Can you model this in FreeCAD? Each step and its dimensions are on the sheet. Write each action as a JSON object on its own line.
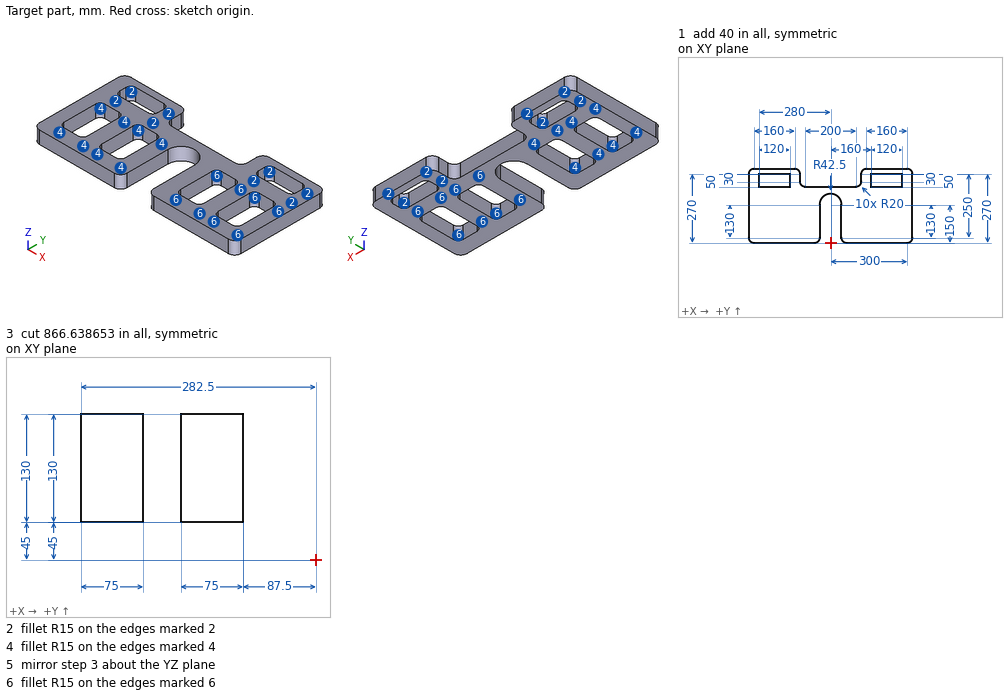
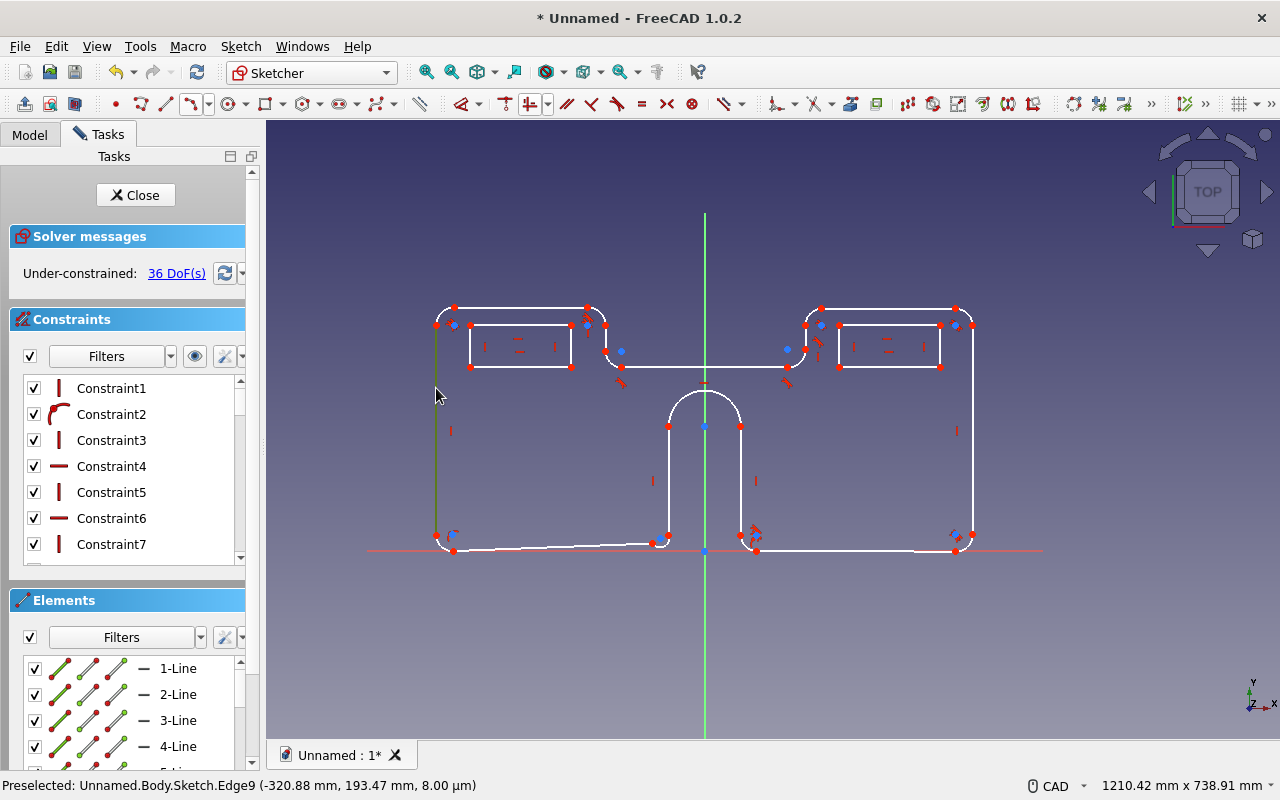
{"action": "scroll", "coordinate": [438, 543], "scroll_direction": "up", "scroll_amount": 3}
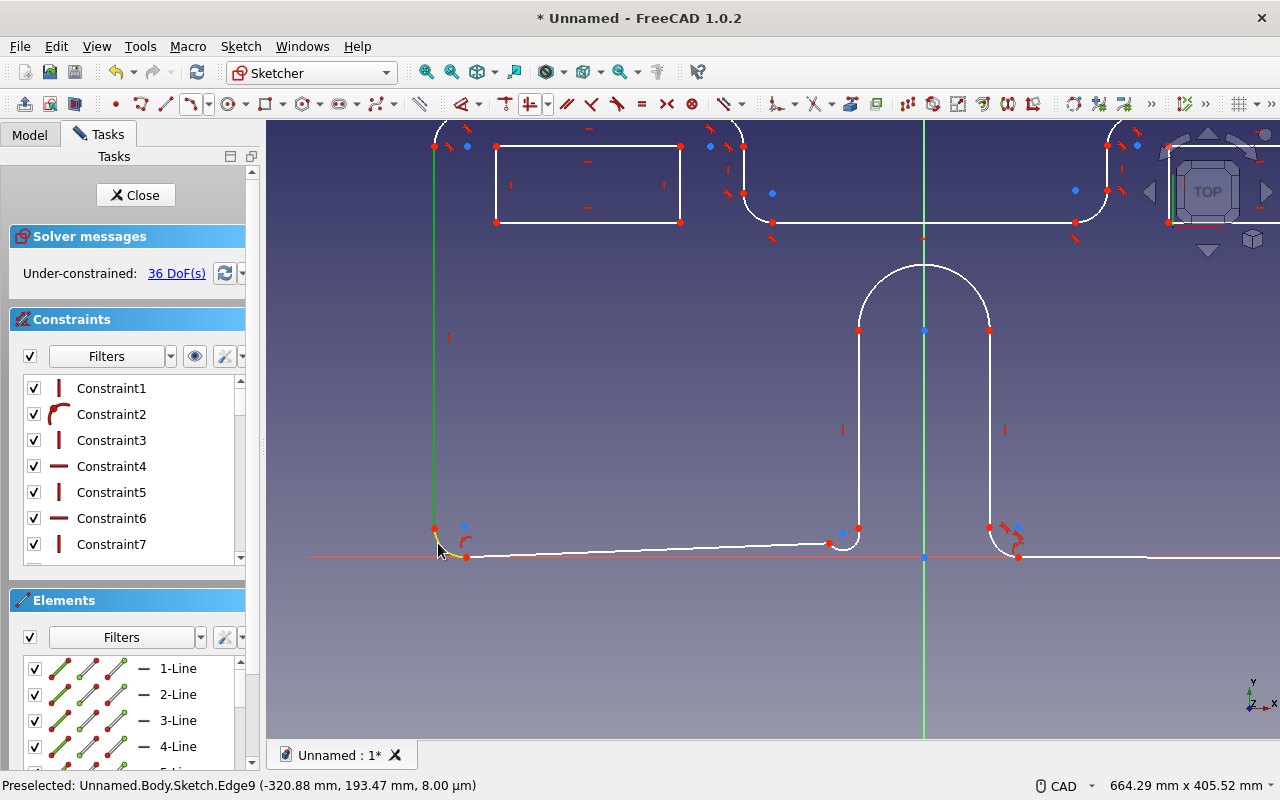
{"action": "left_click", "coordinate": [439, 542]}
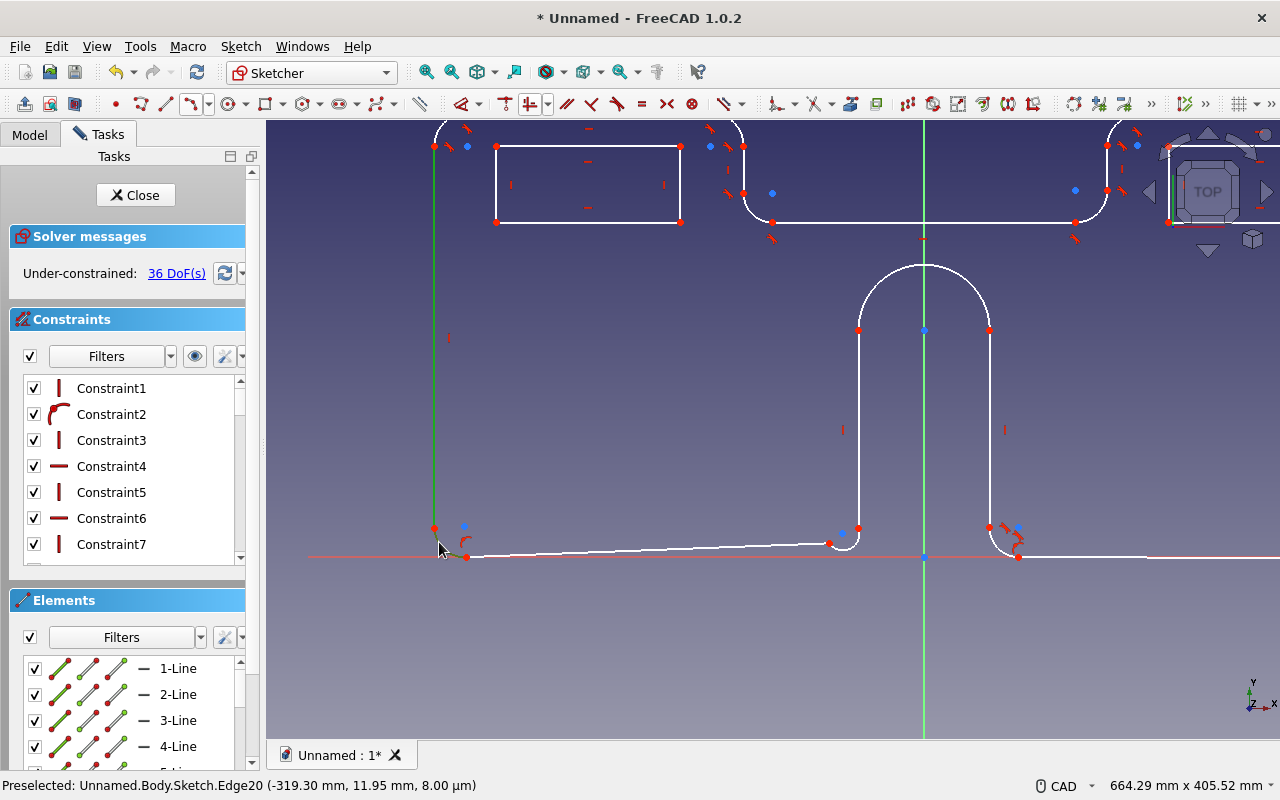
{"action": "left_click", "coordinate": [617, 104]}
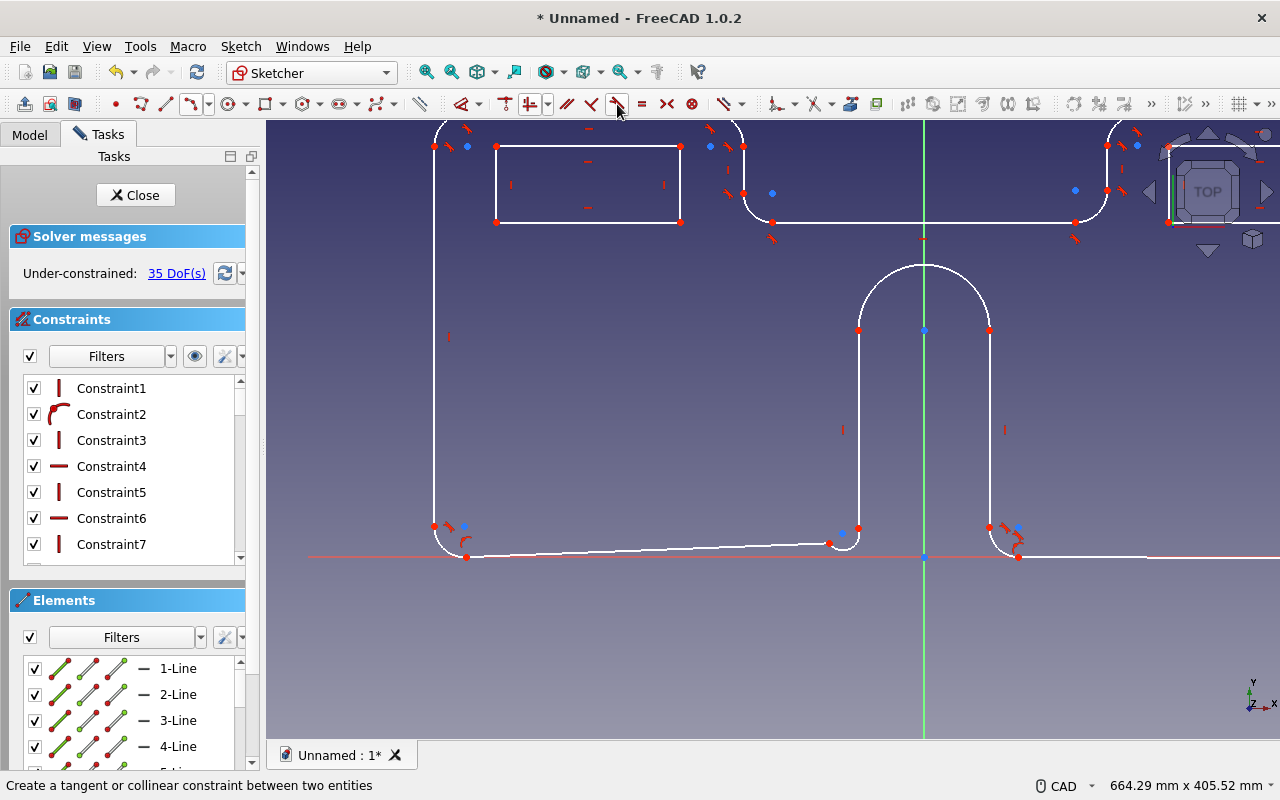
{"action": "scroll", "coordinate": [721, 547], "scroll_direction": "up", "scroll_amount": 2}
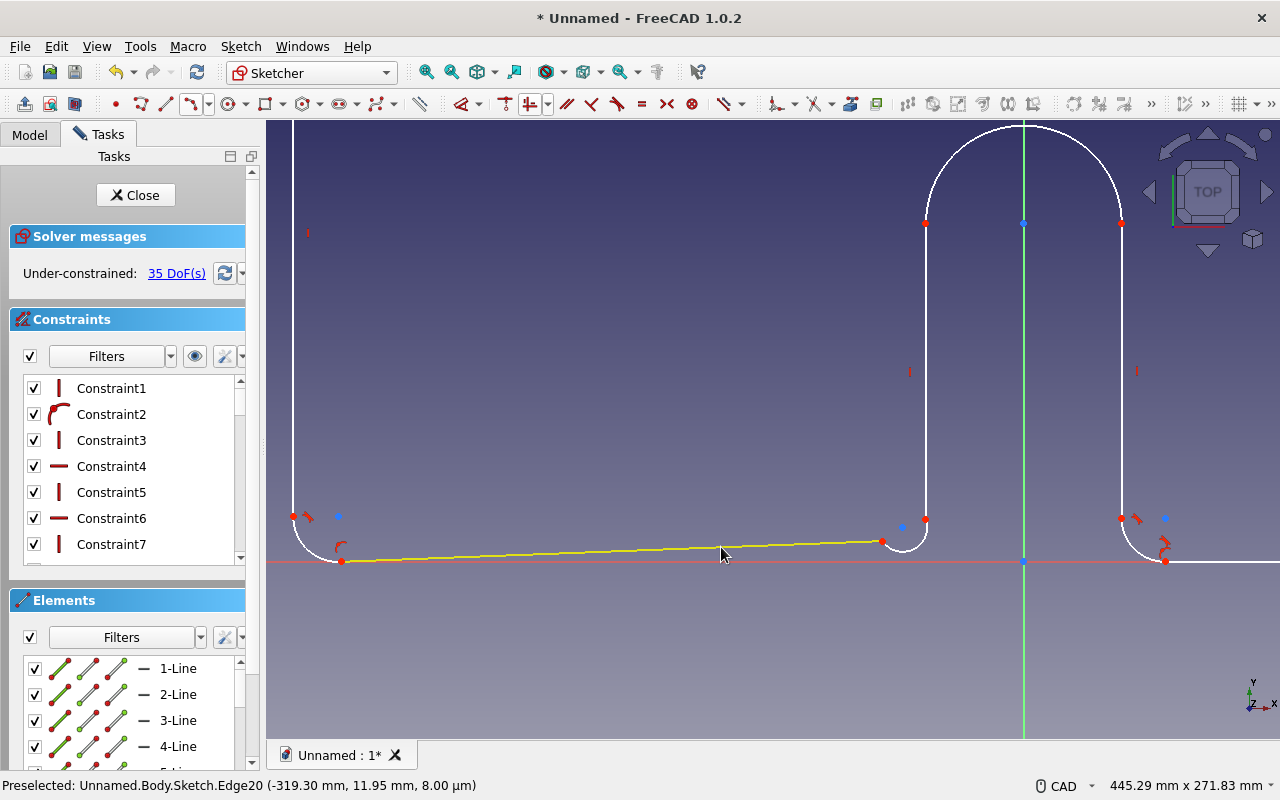
{"action": "left_click", "coordinate": [720, 547]}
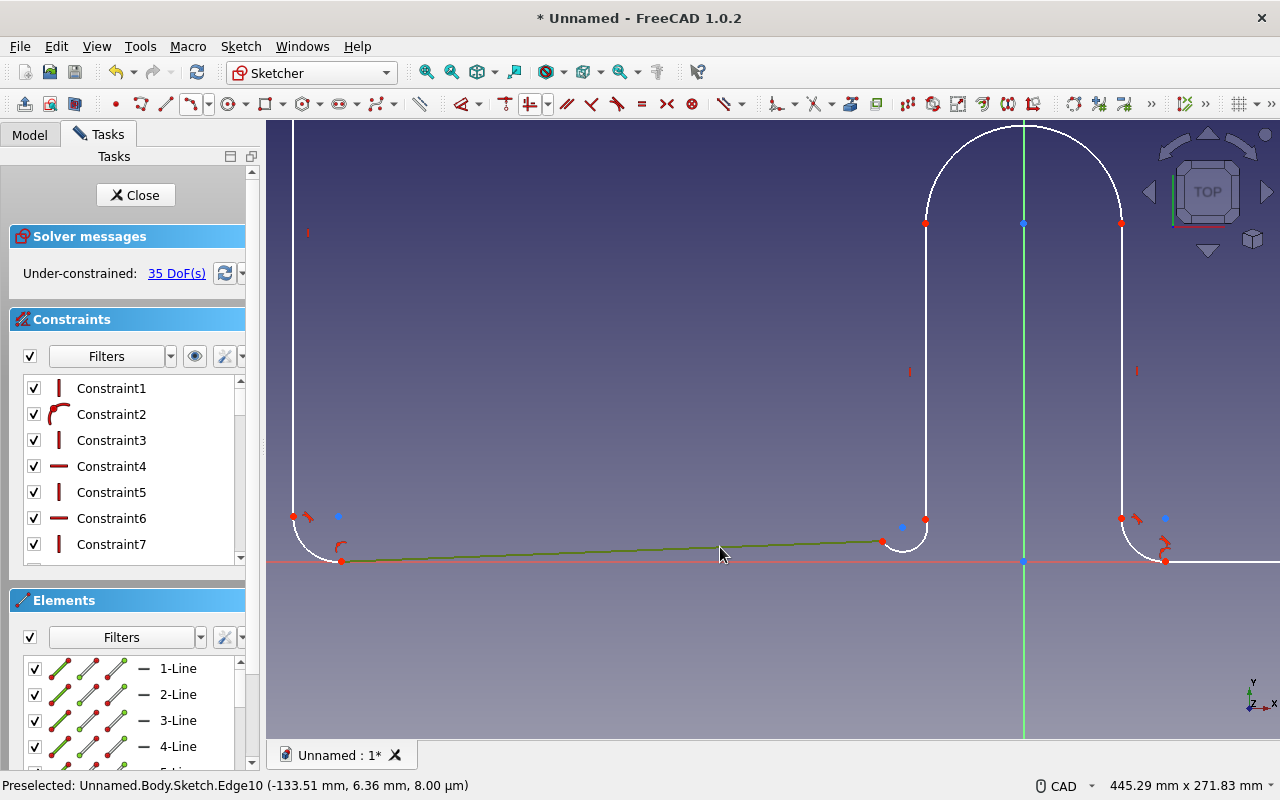
{"action": "left_click", "coordinate": [299, 538]}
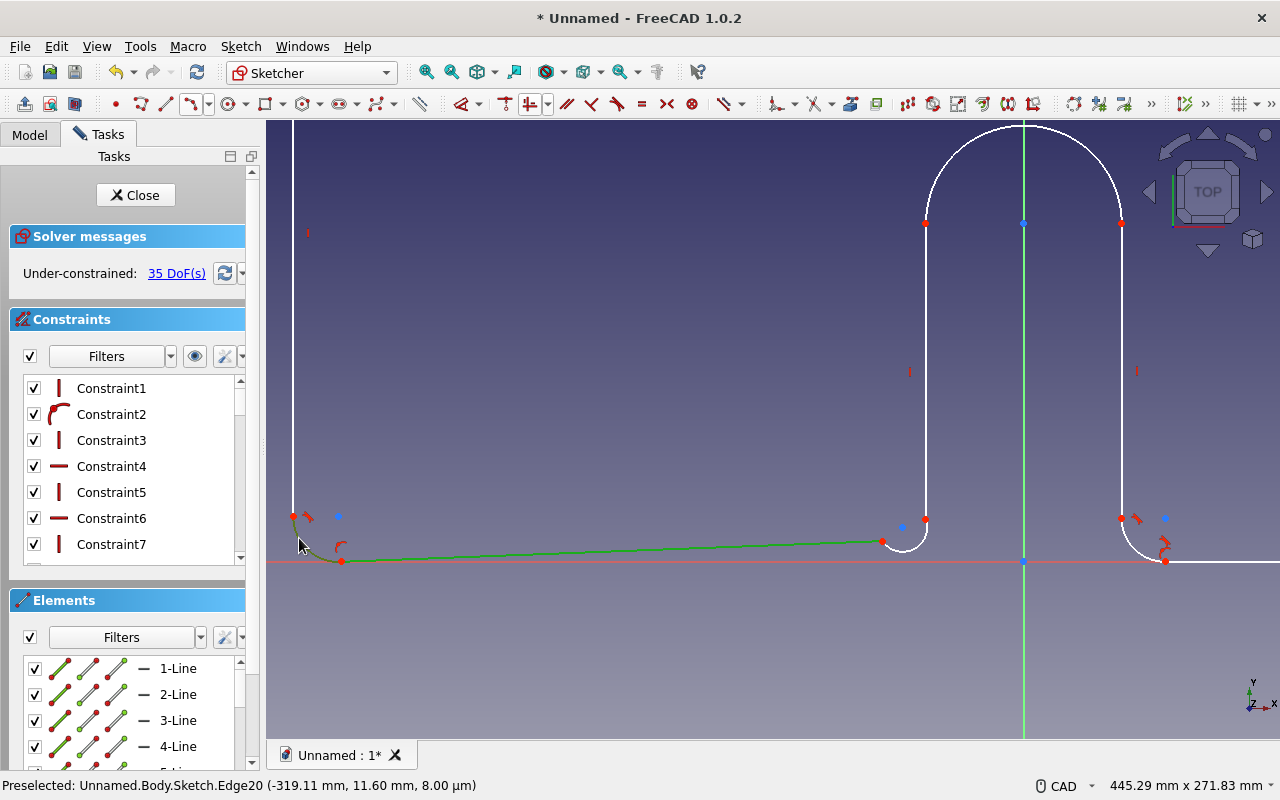
{"action": "key", "text": "t"}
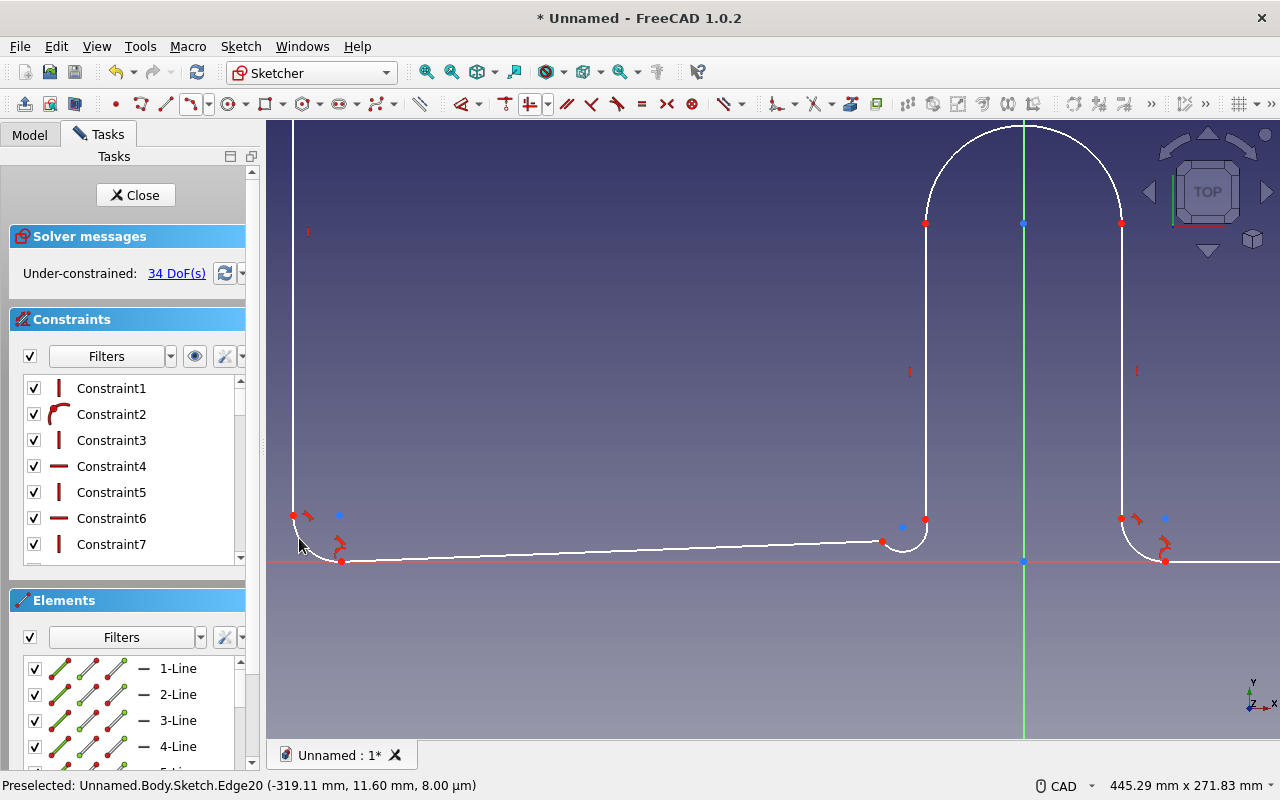
{"action": "left_click", "coordinate": [720, 547]}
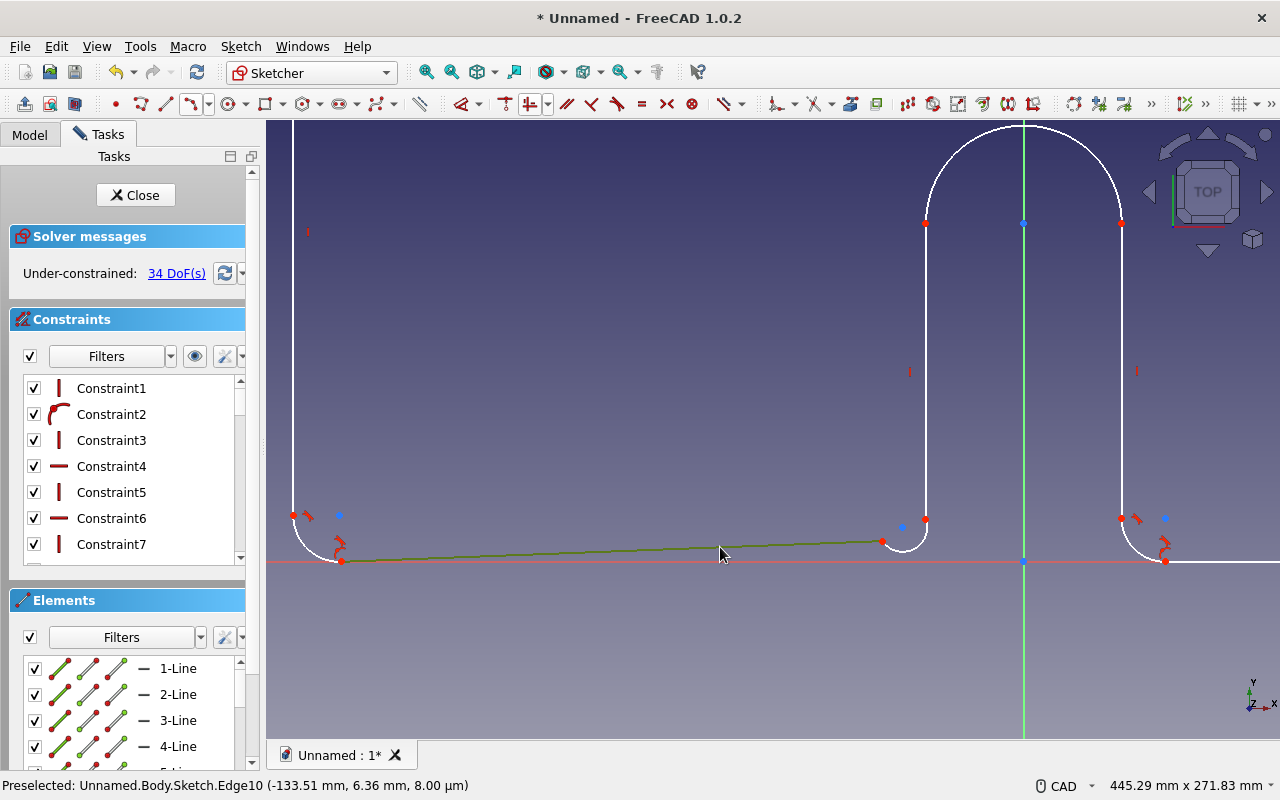
{"action": "scroll", "coordinate": [900, 552], "scroll_direction": "up", "scroll_amount": 2}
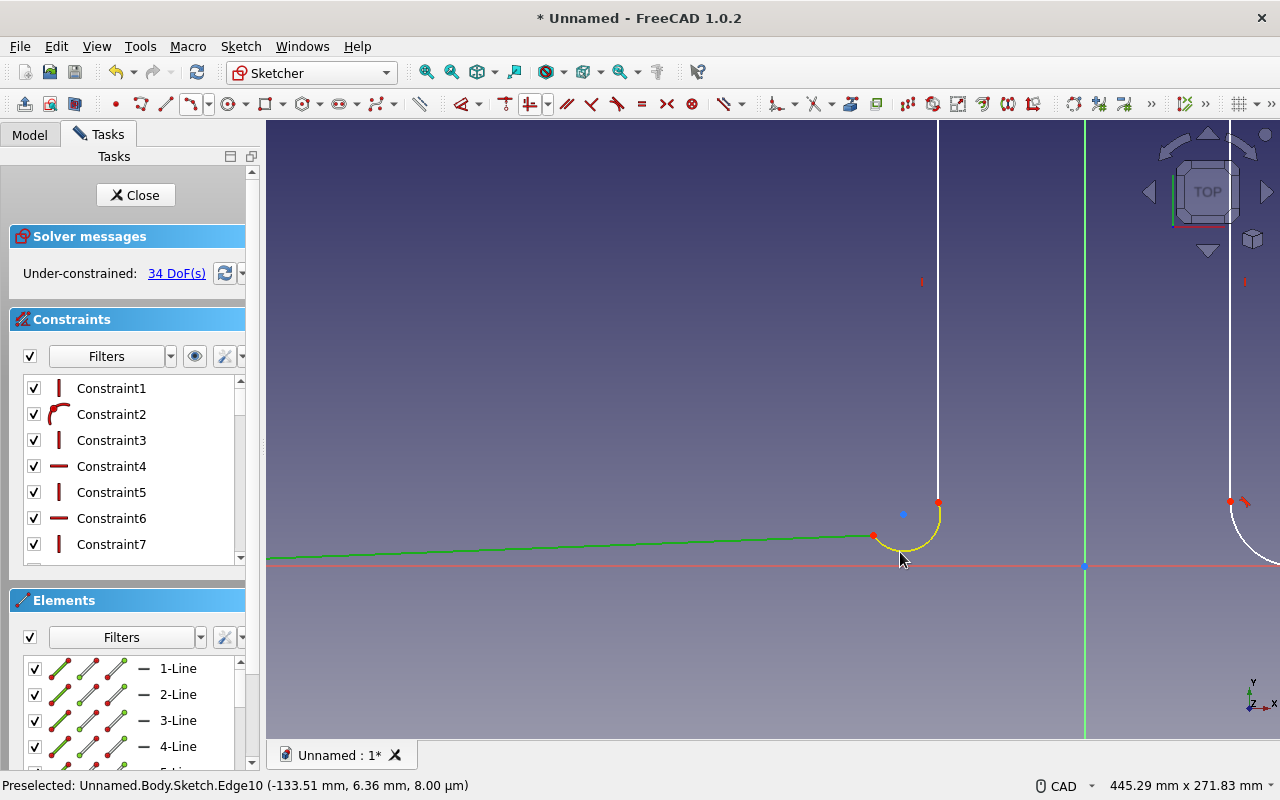
{"action": "left_click", "coordinate": [900, 551]}